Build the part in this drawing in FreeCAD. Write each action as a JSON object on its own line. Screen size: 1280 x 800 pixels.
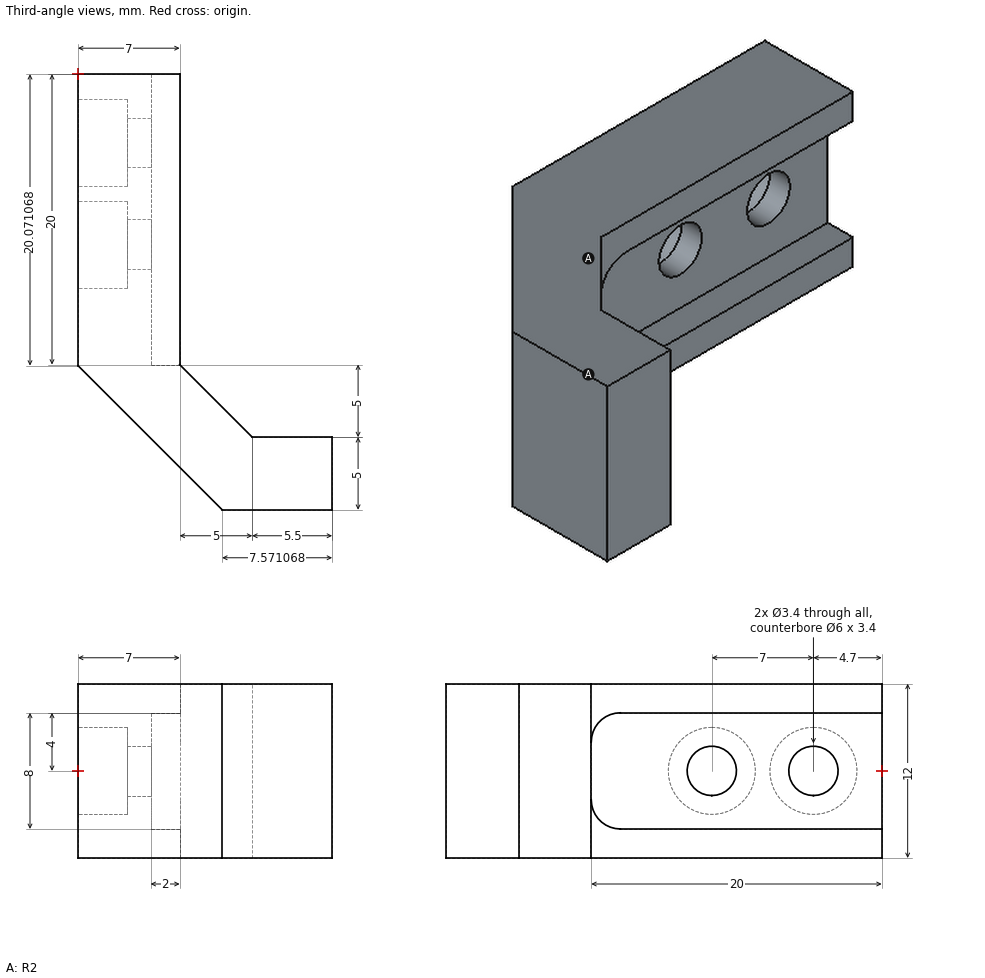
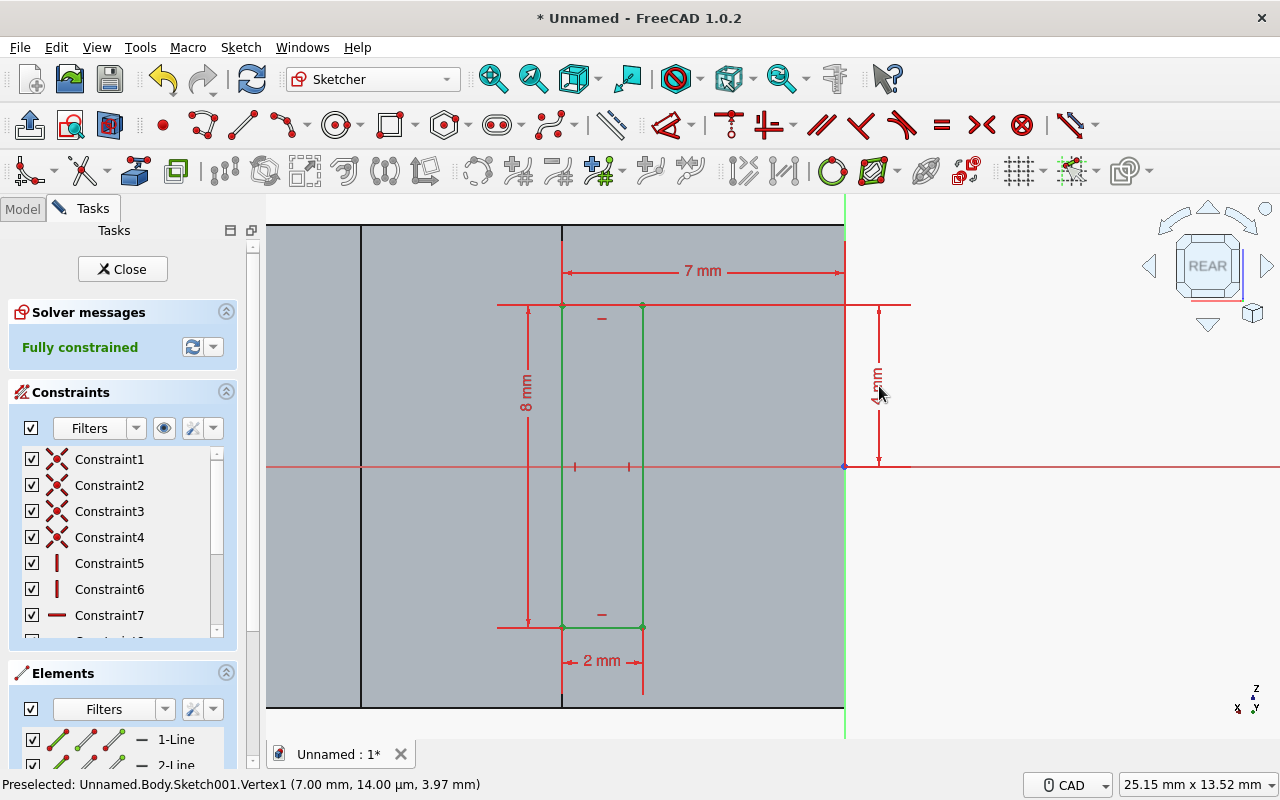
{"action": "left_click", "coordinate": [123, 269]}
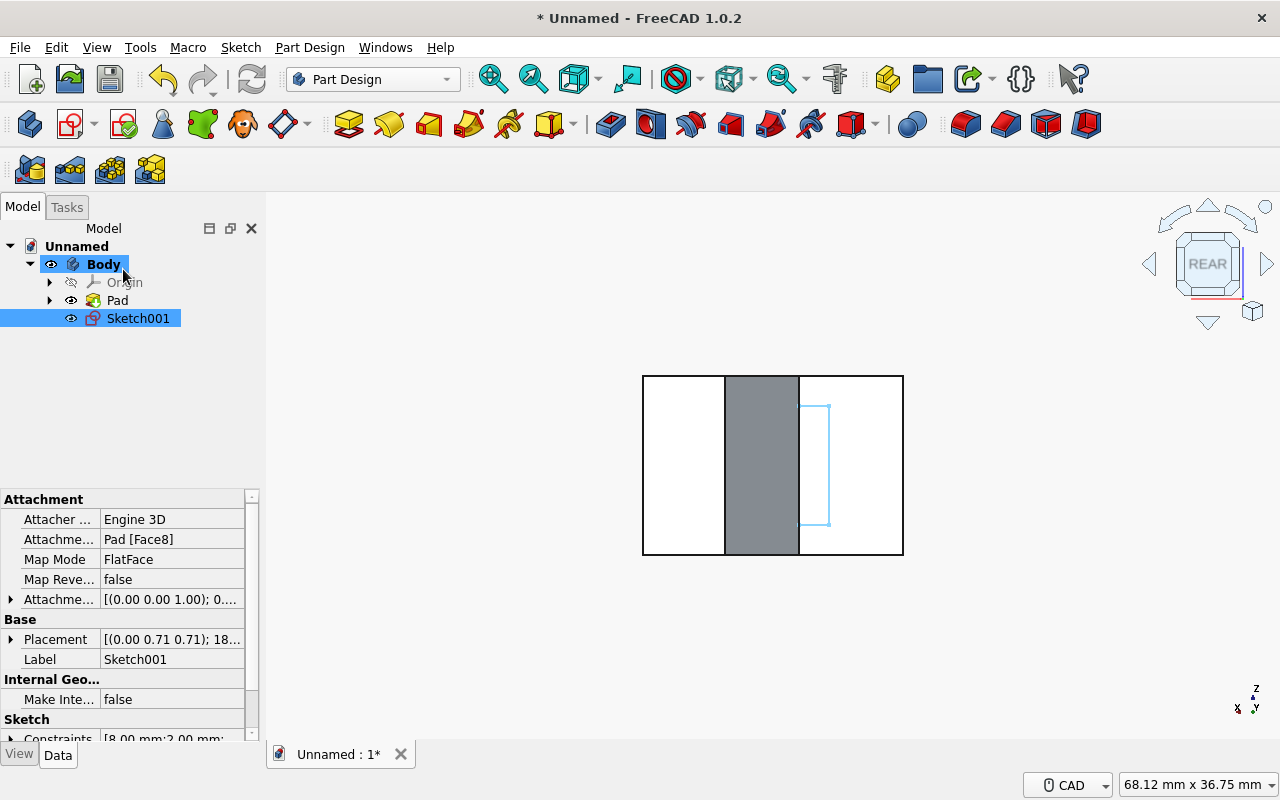
{"action": "left_click", "coordinate": [612, 124]}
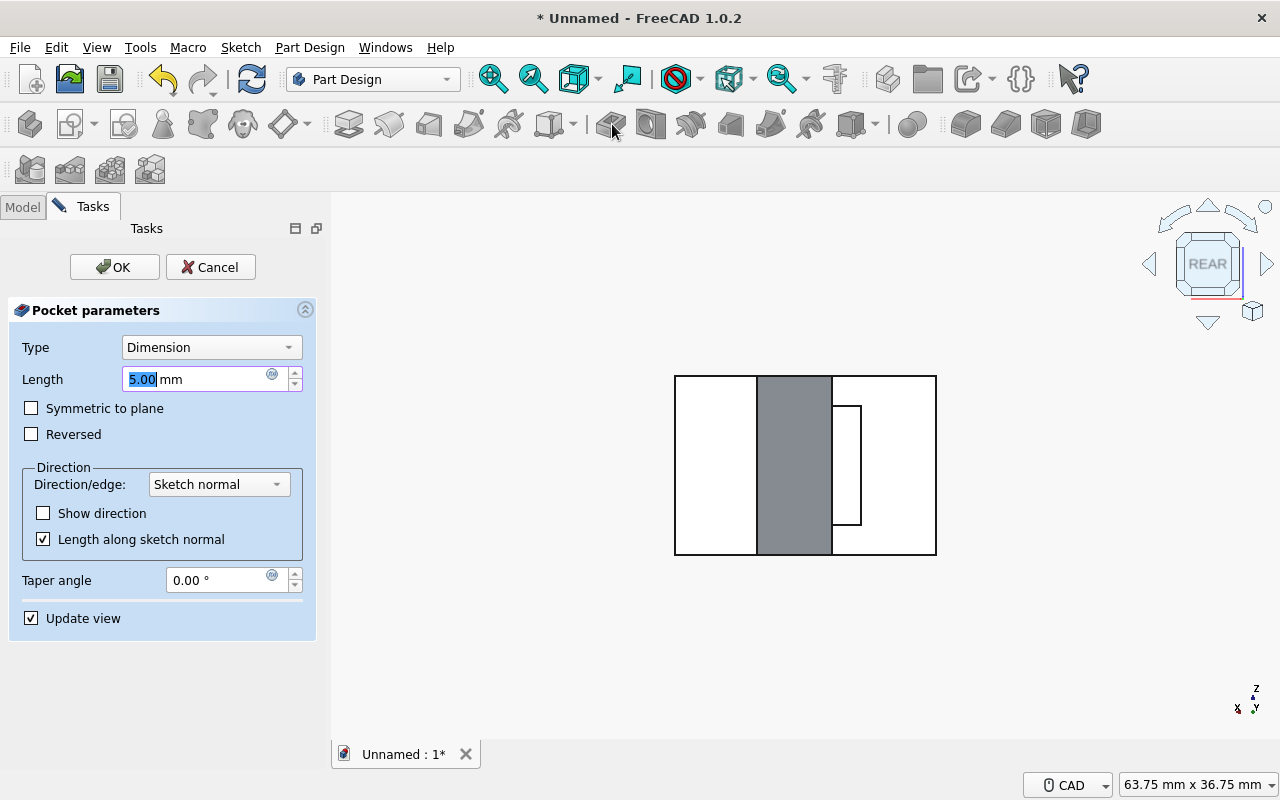
{"action": "type", "text": "20"}
{"action": "key", "text": "Tab"}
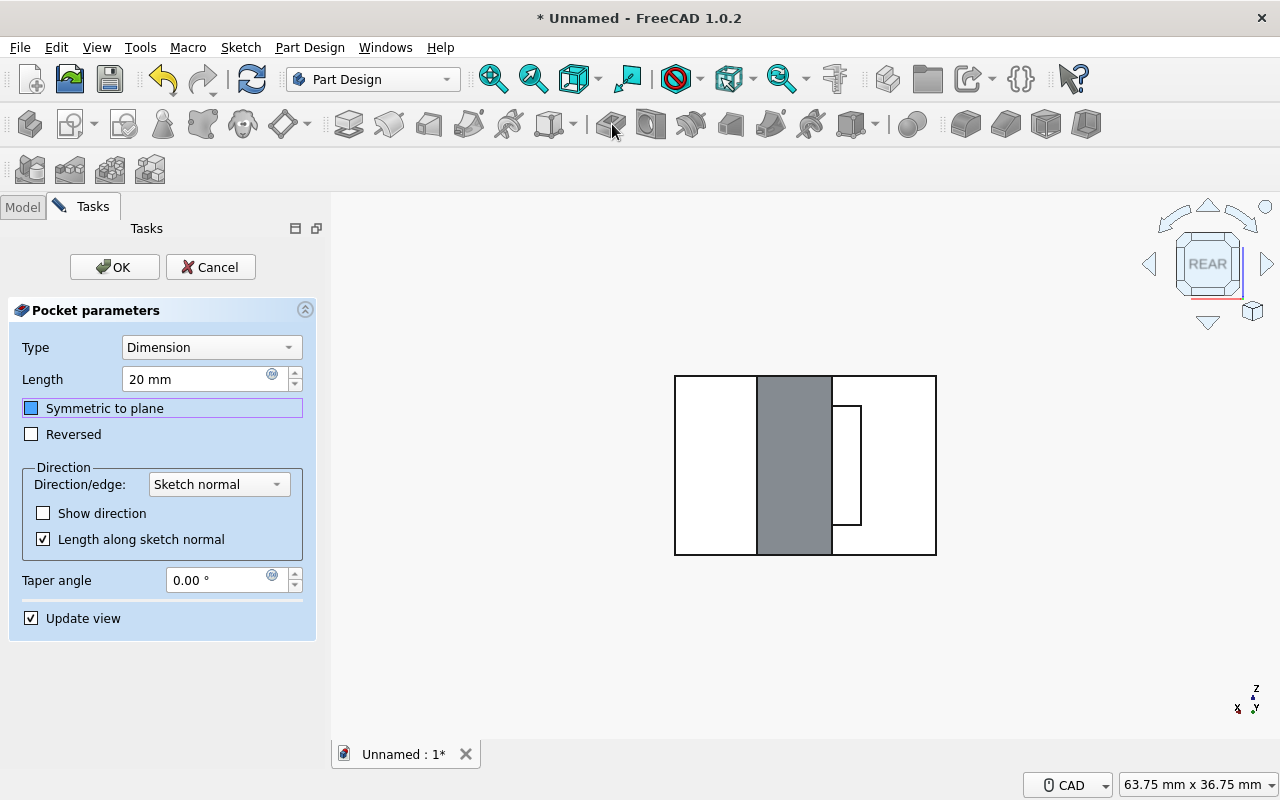
{"action": "left_click", "coordinate": [115, 267]}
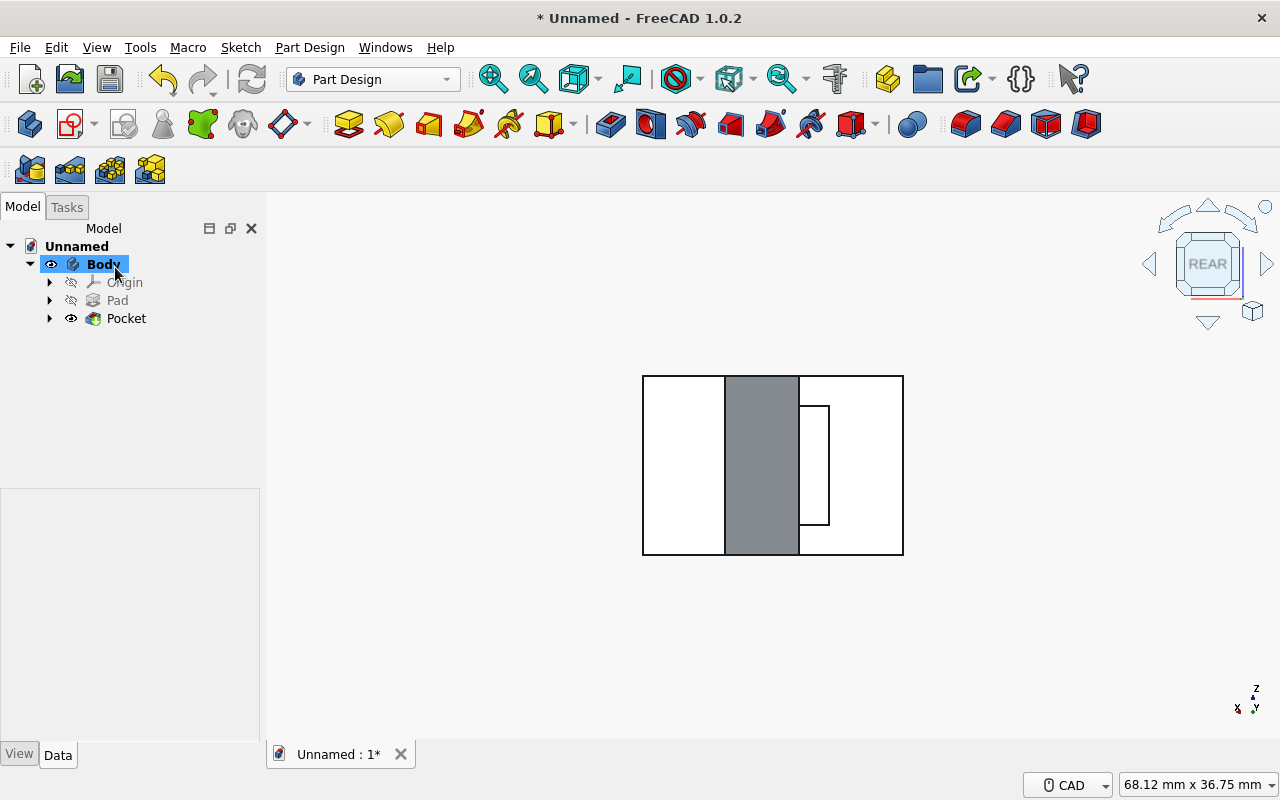
{"action": "left_click", "coordinate": [494, 80]}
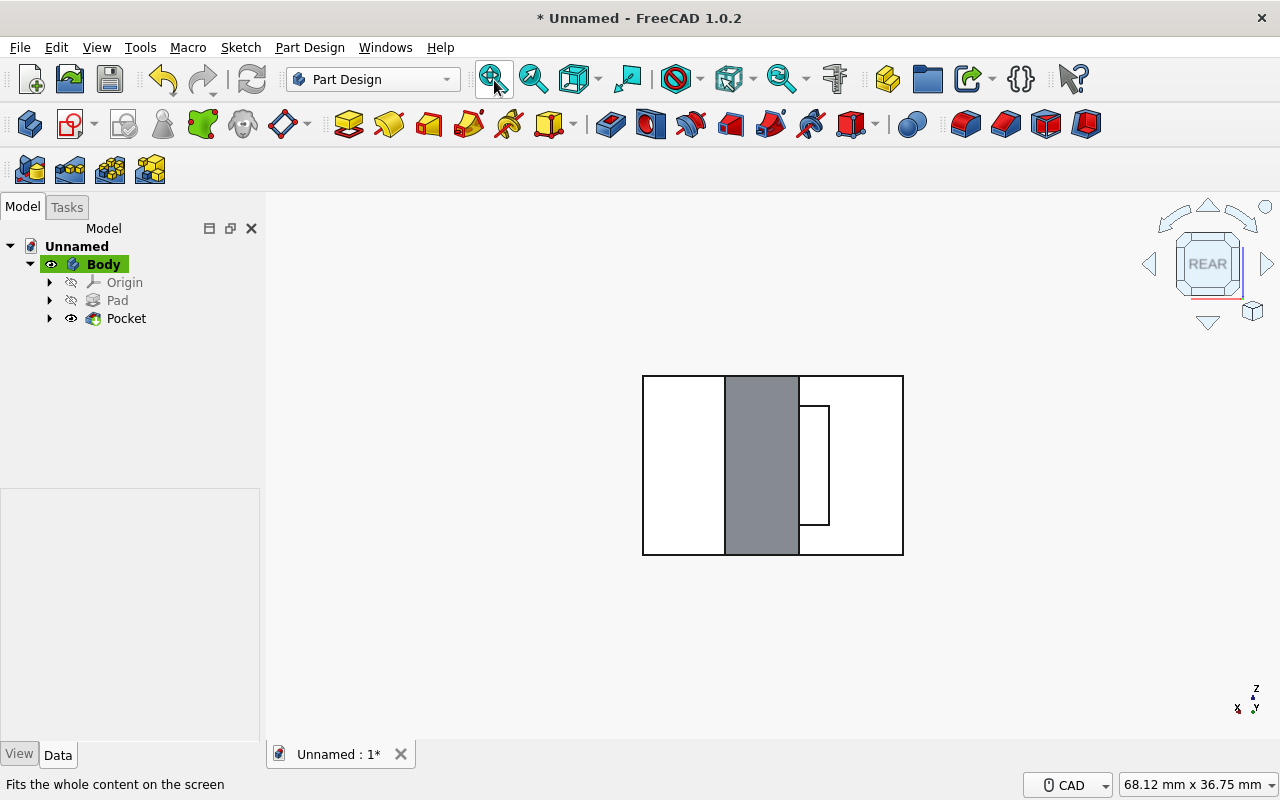
{"action": "key", "text": "0"}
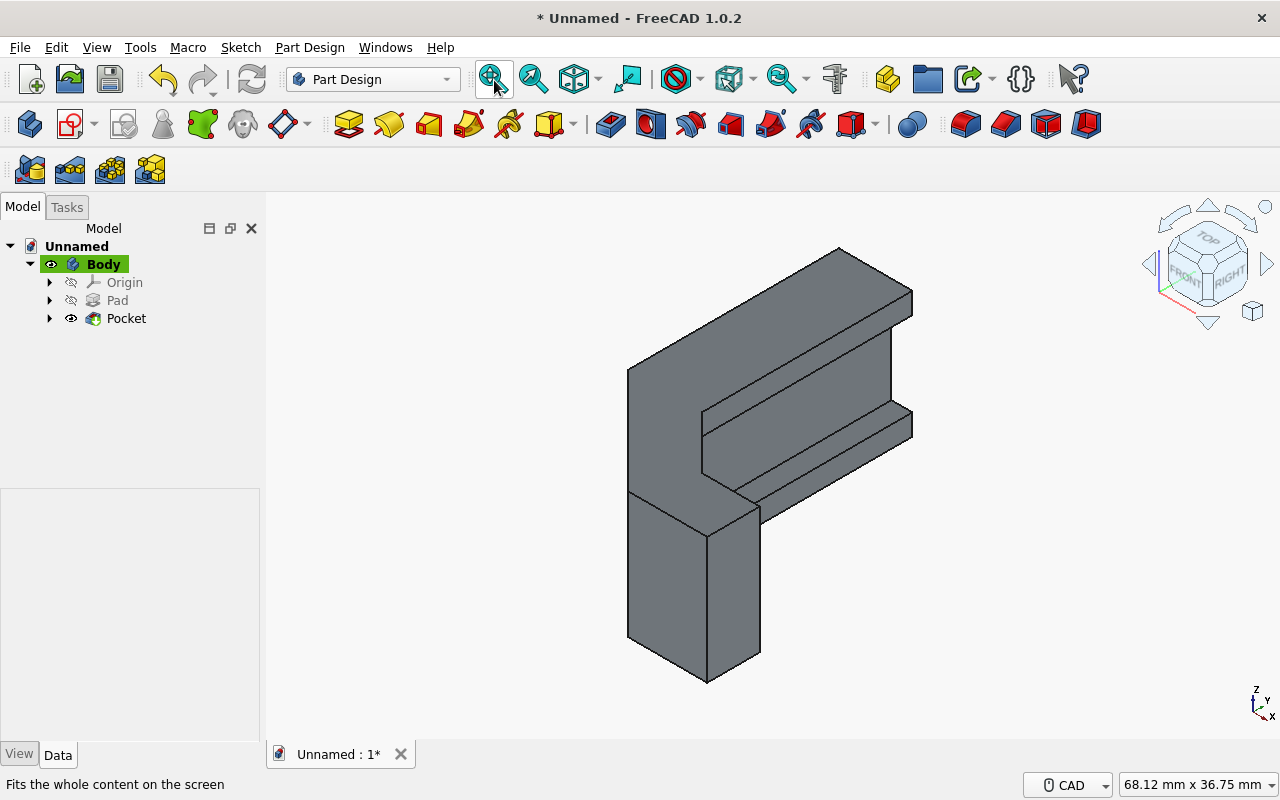
{"action": "key", "text": "2"}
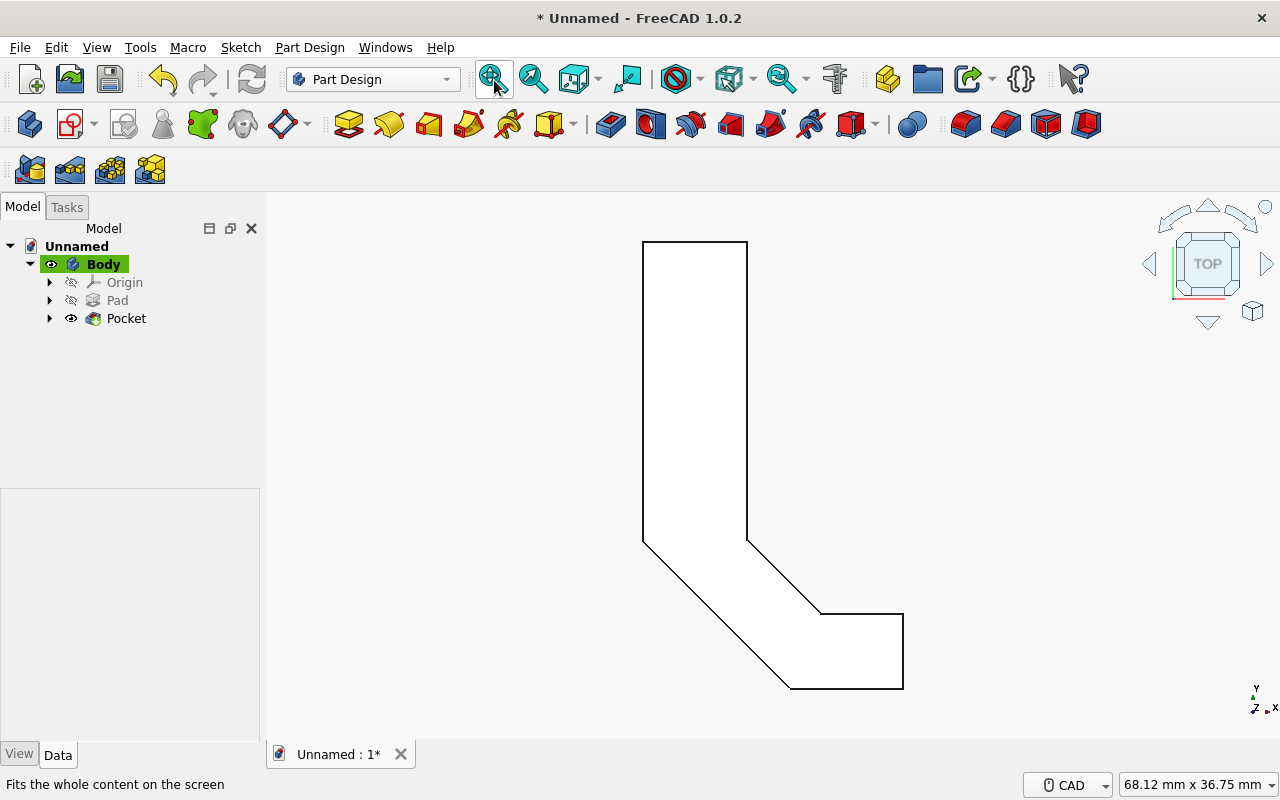
{"action": "key", "text": "1"}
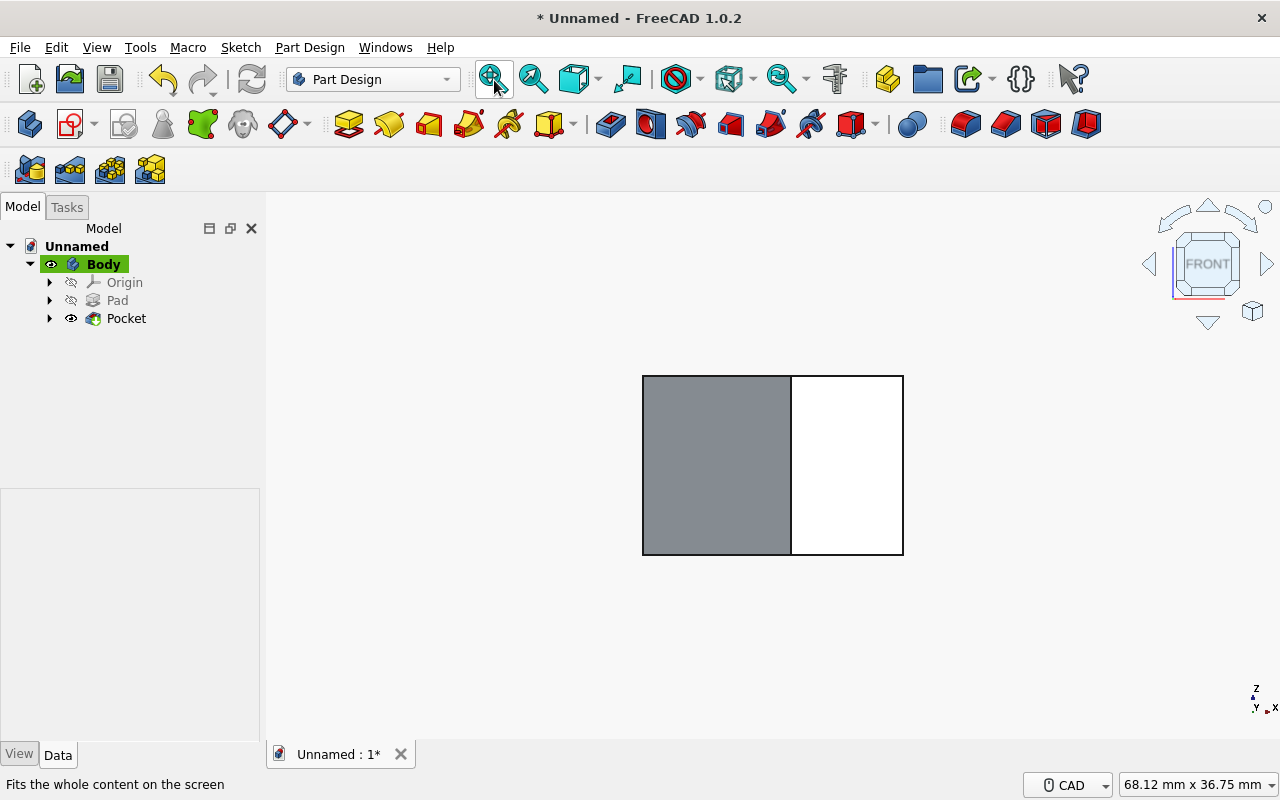
{"action": "left_click", "coordinate": [494, 80]}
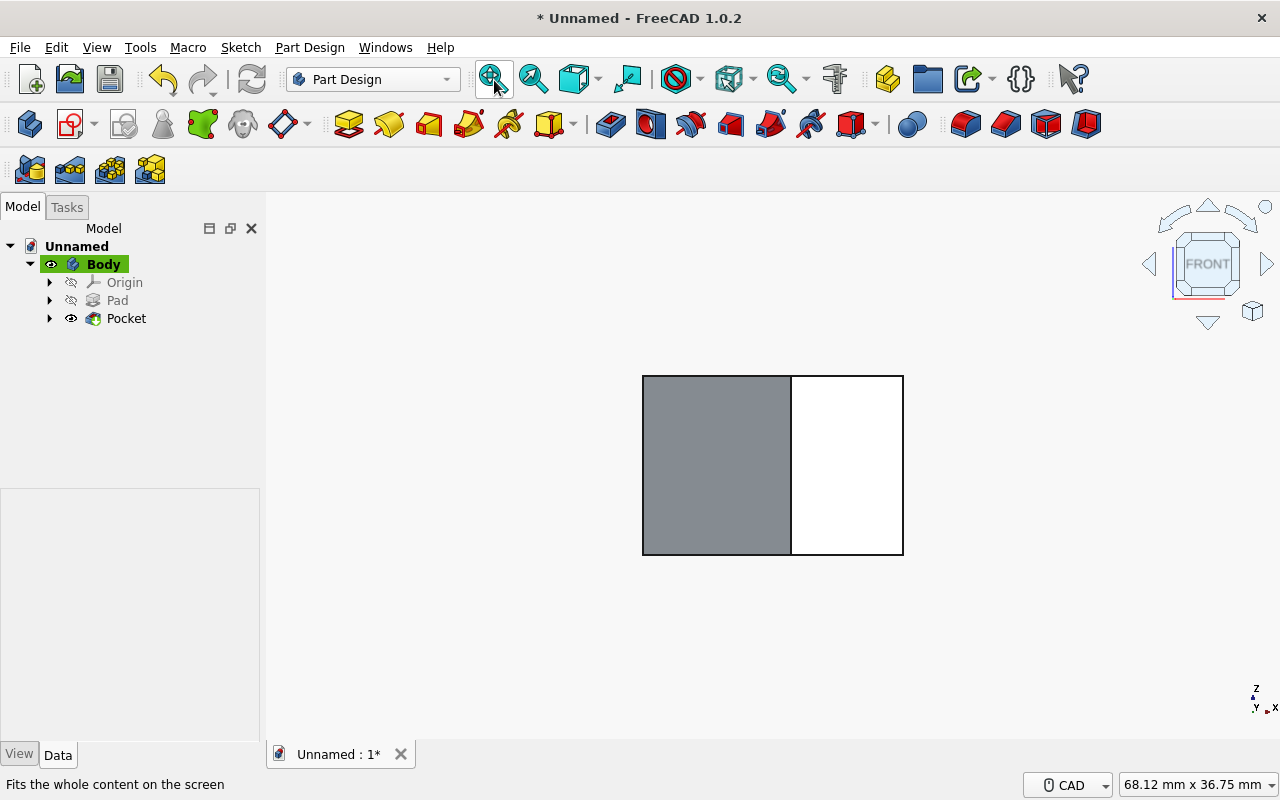
{"action": "key", "text": "3"}